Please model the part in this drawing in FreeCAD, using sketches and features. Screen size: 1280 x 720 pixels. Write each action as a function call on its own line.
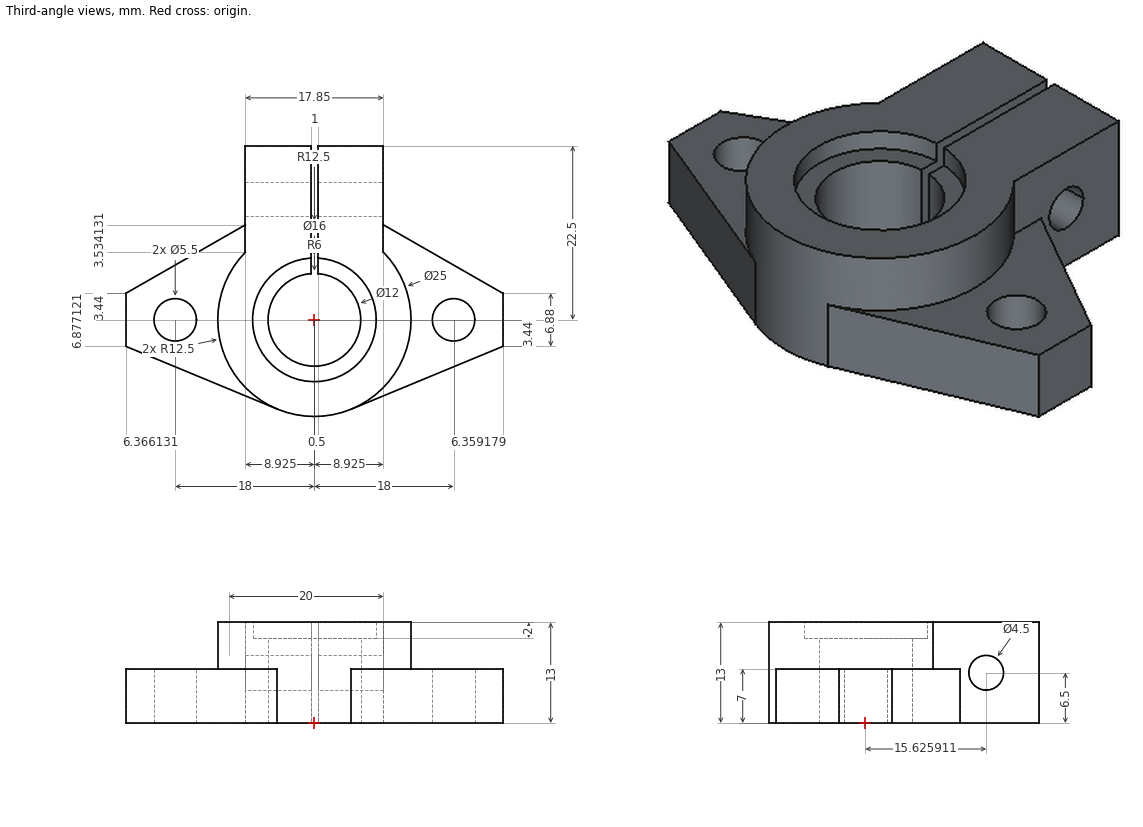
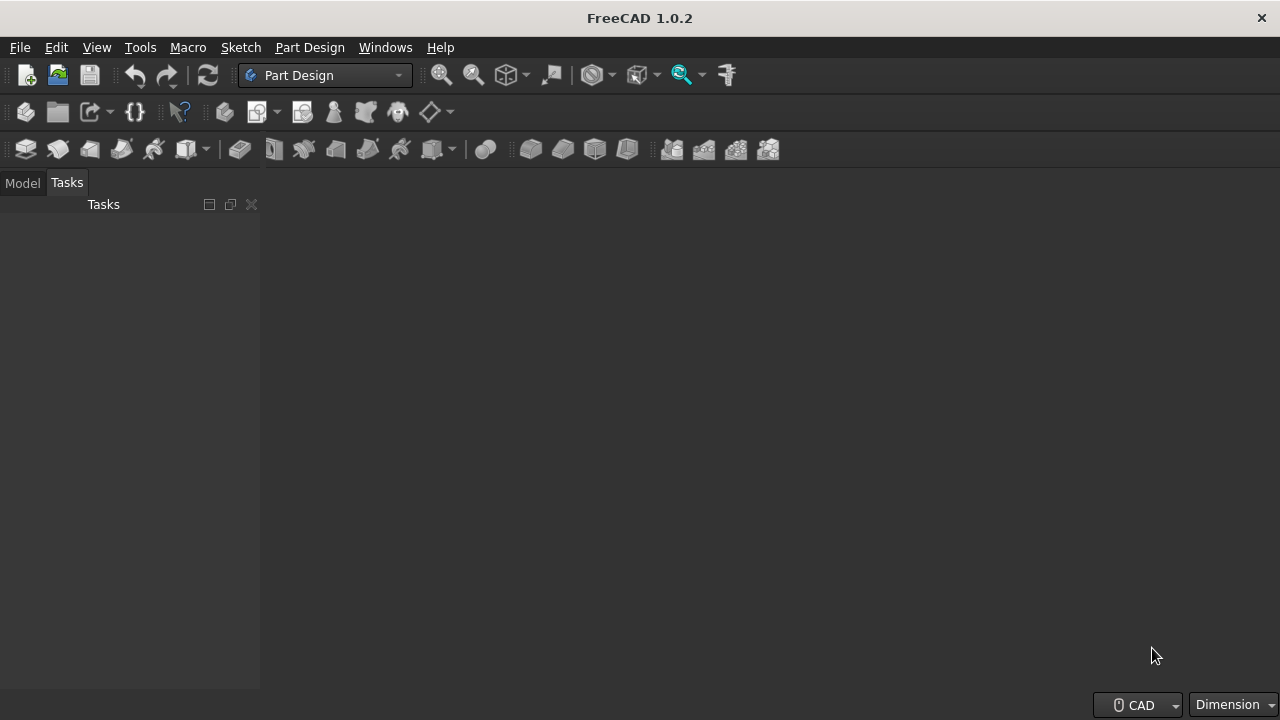
click(26, 76)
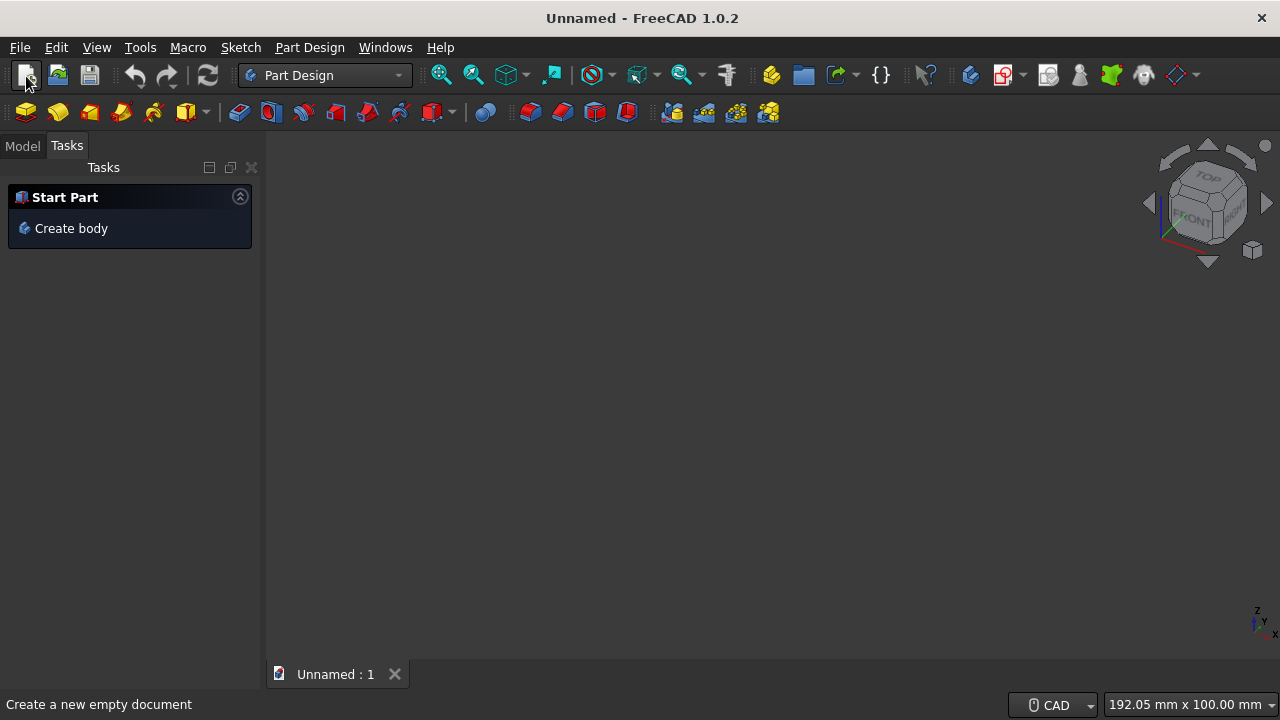
click(1004, 76)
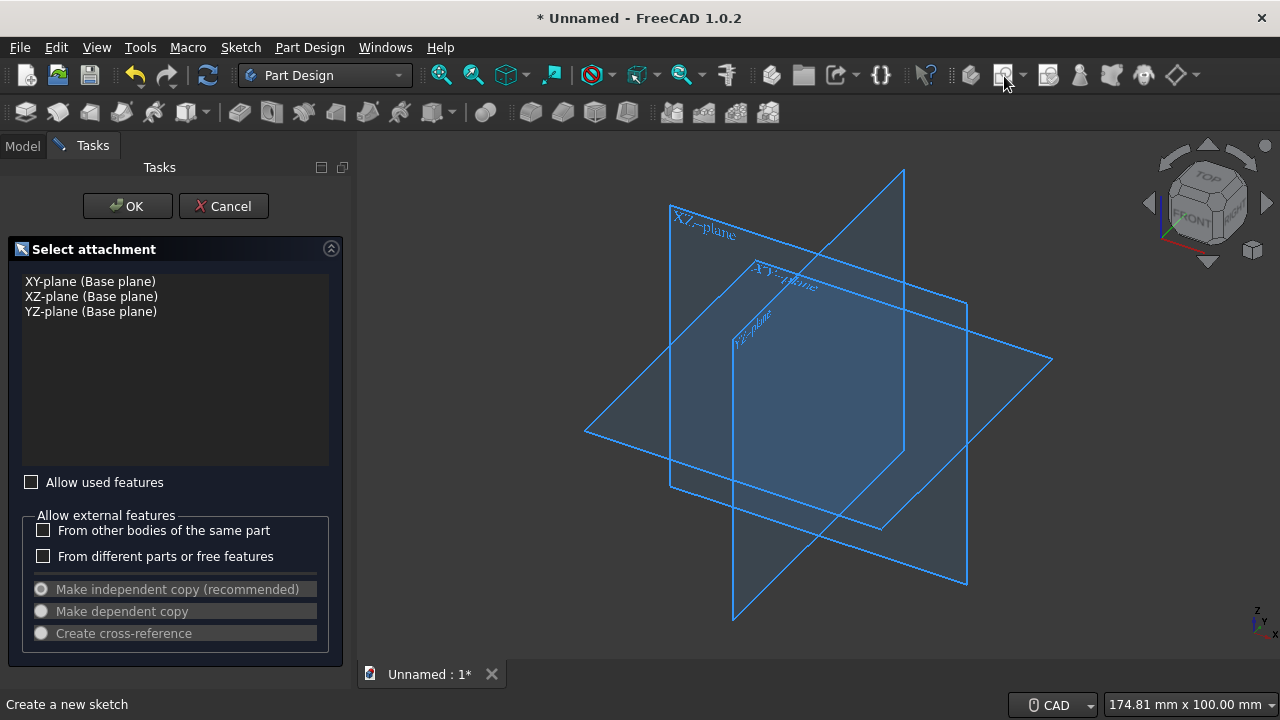
click(82, 282)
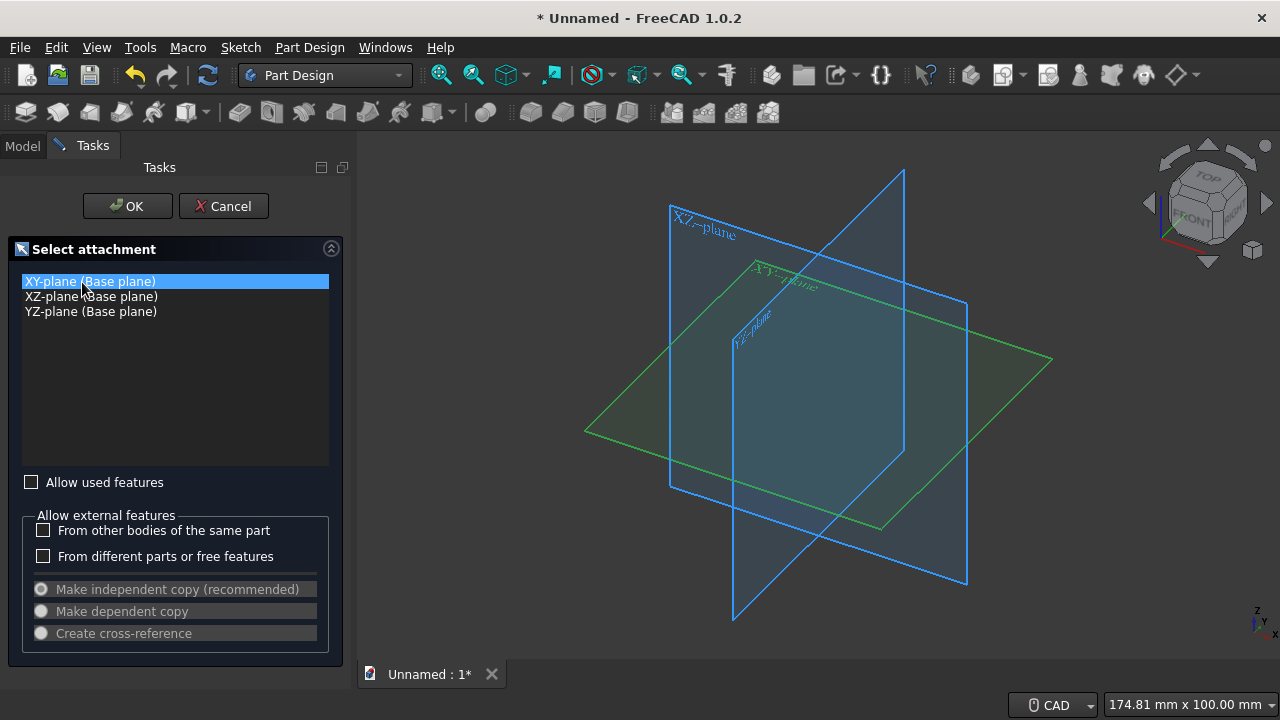
click(128, 206)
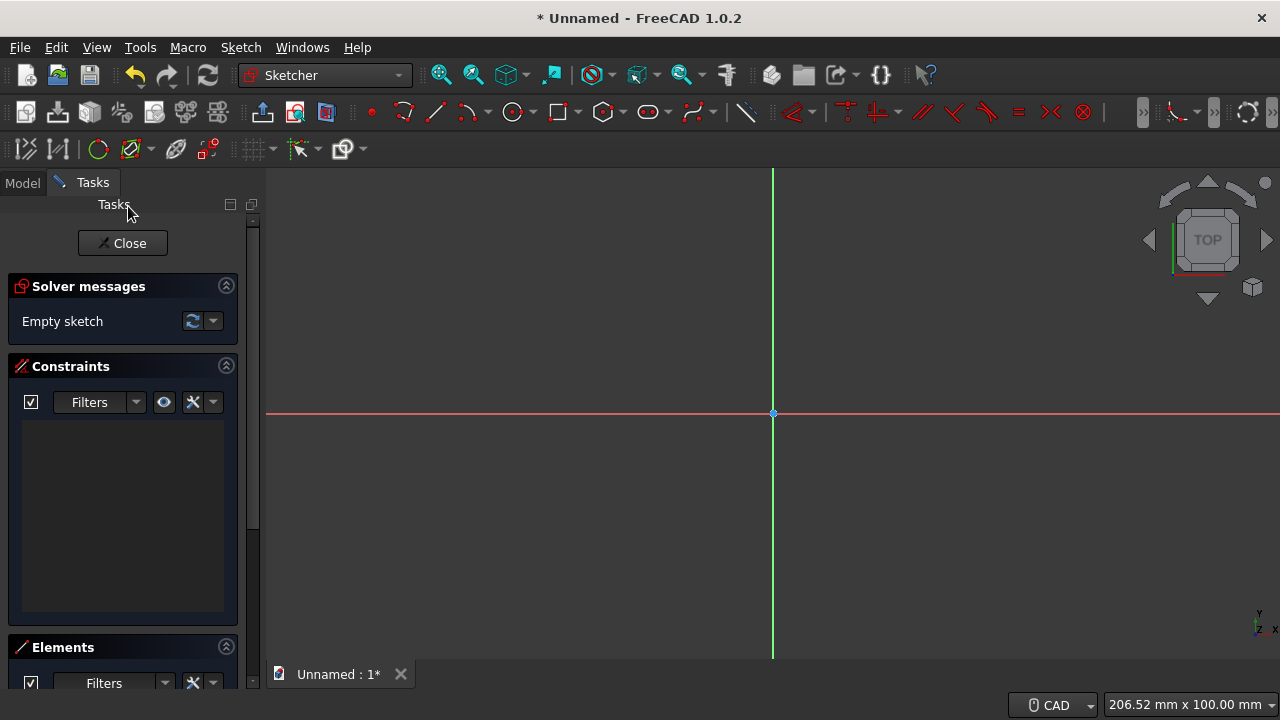
scroll(813, 414, up, 5)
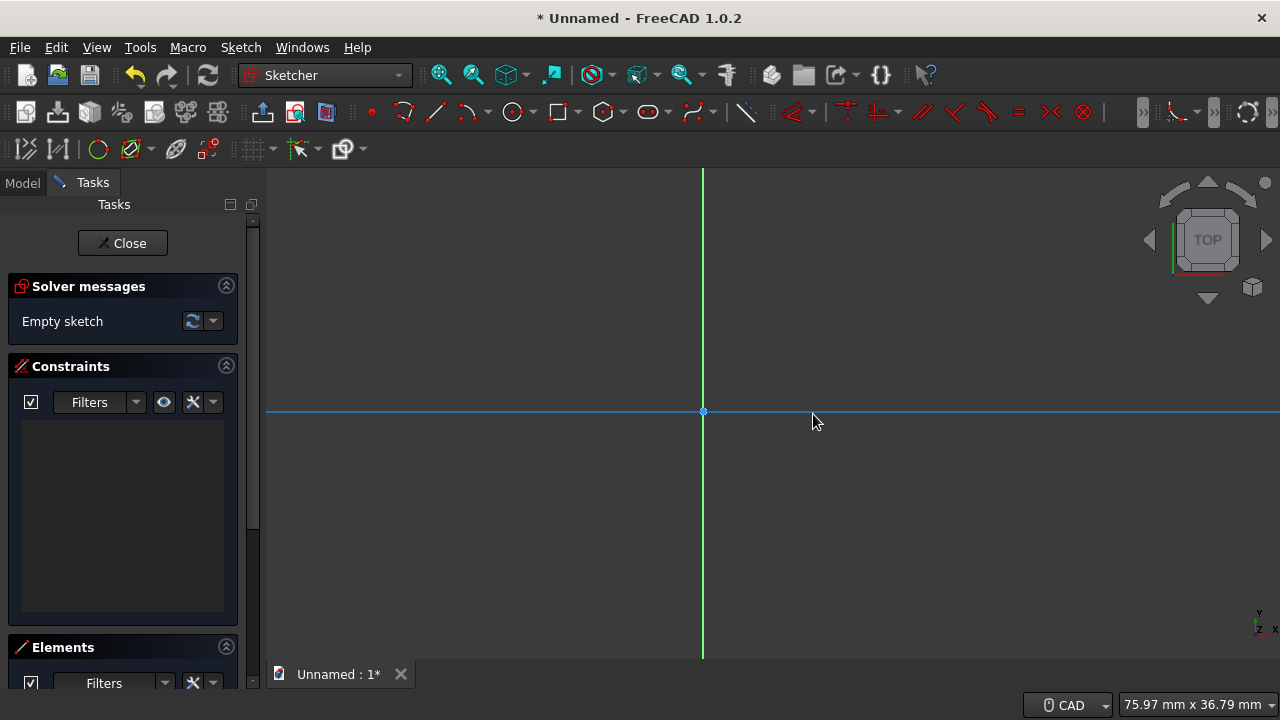
click(514, 112)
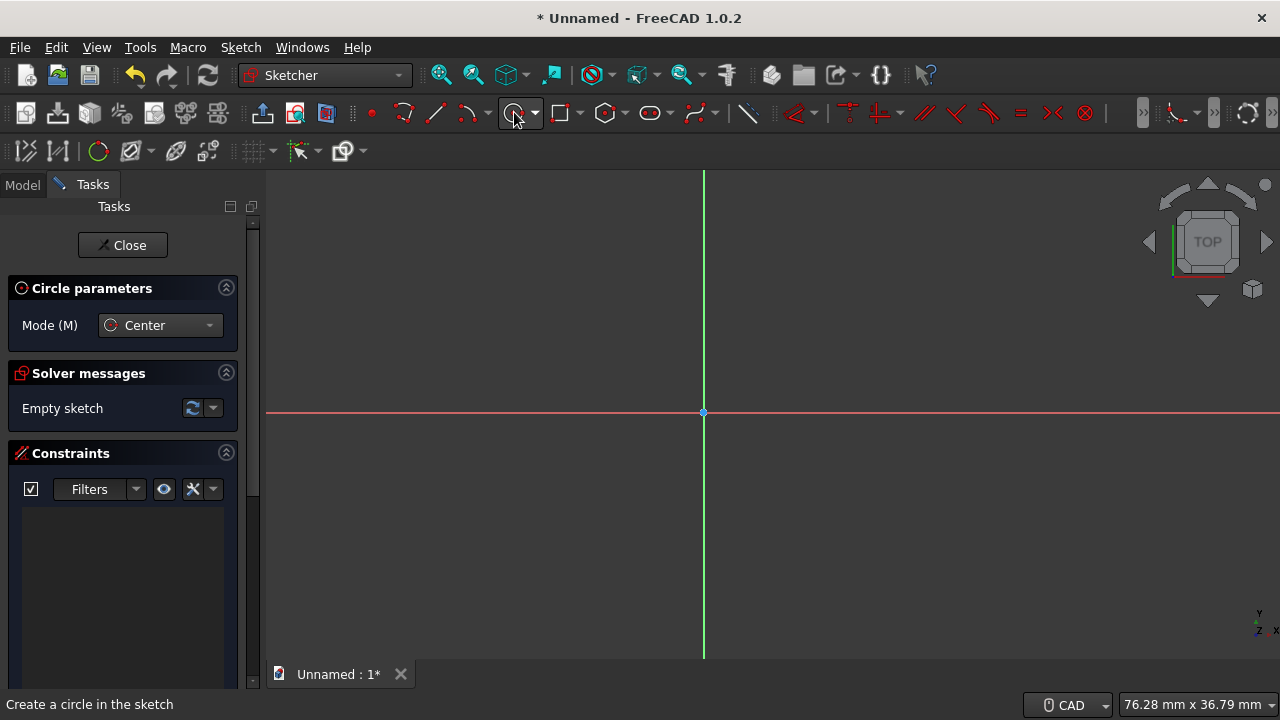
click(704, 413)
click(821, 295)
key(Escape)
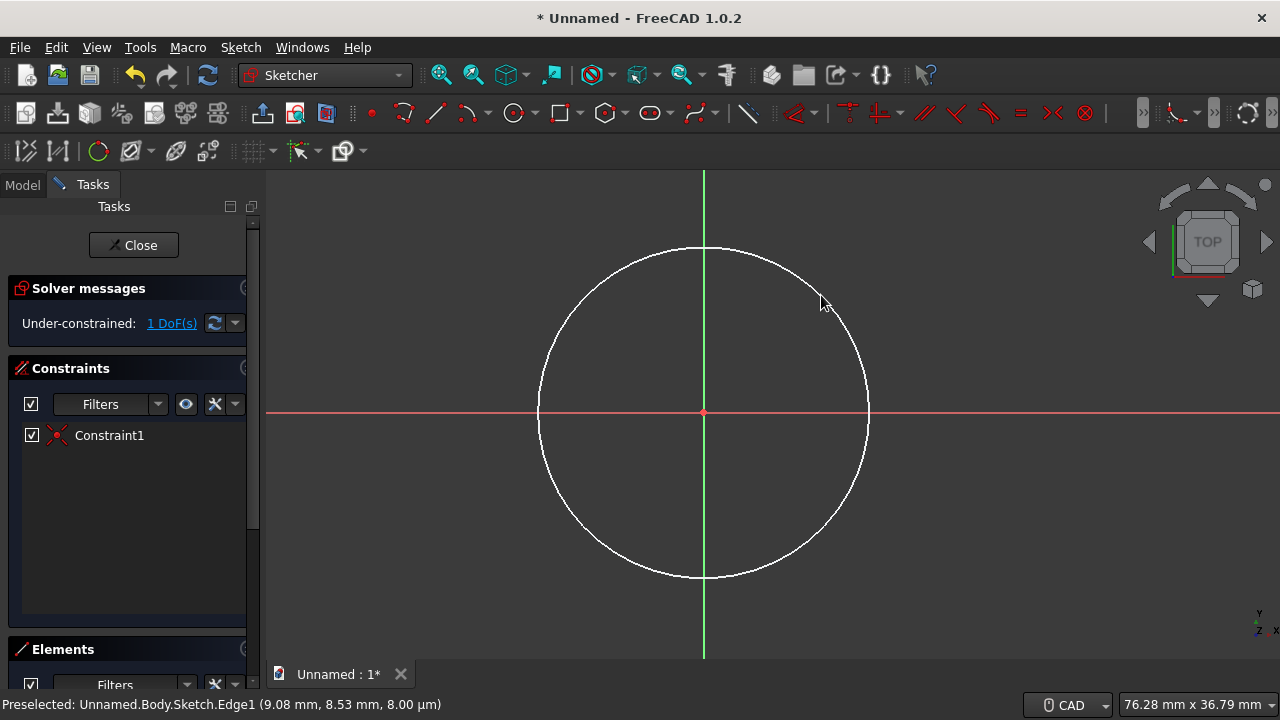
click(820, 295)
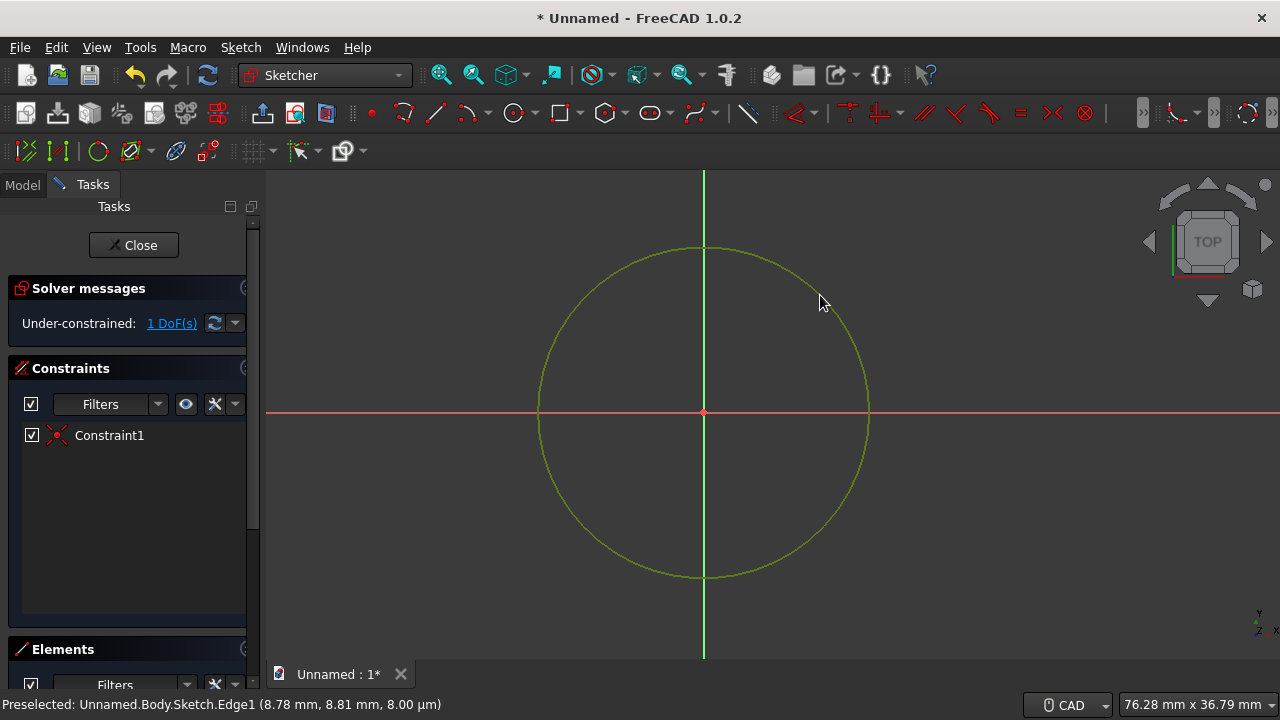
click(816, 114)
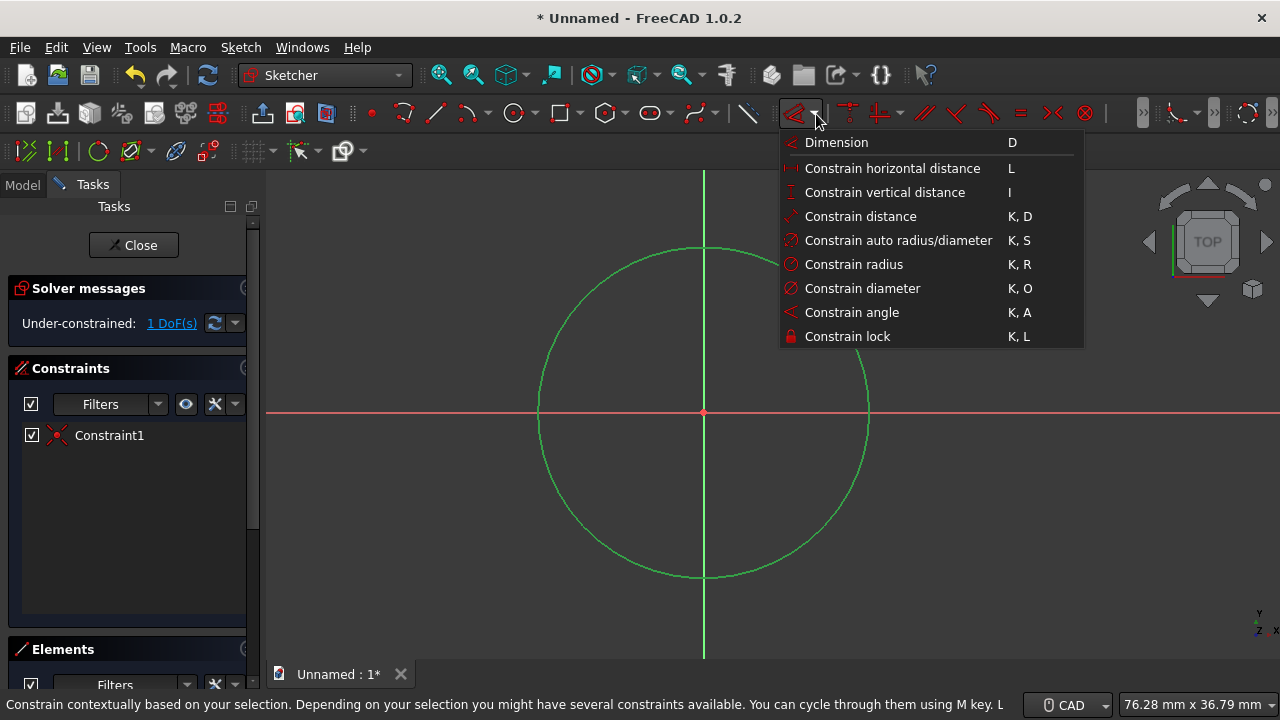
click(932, 288)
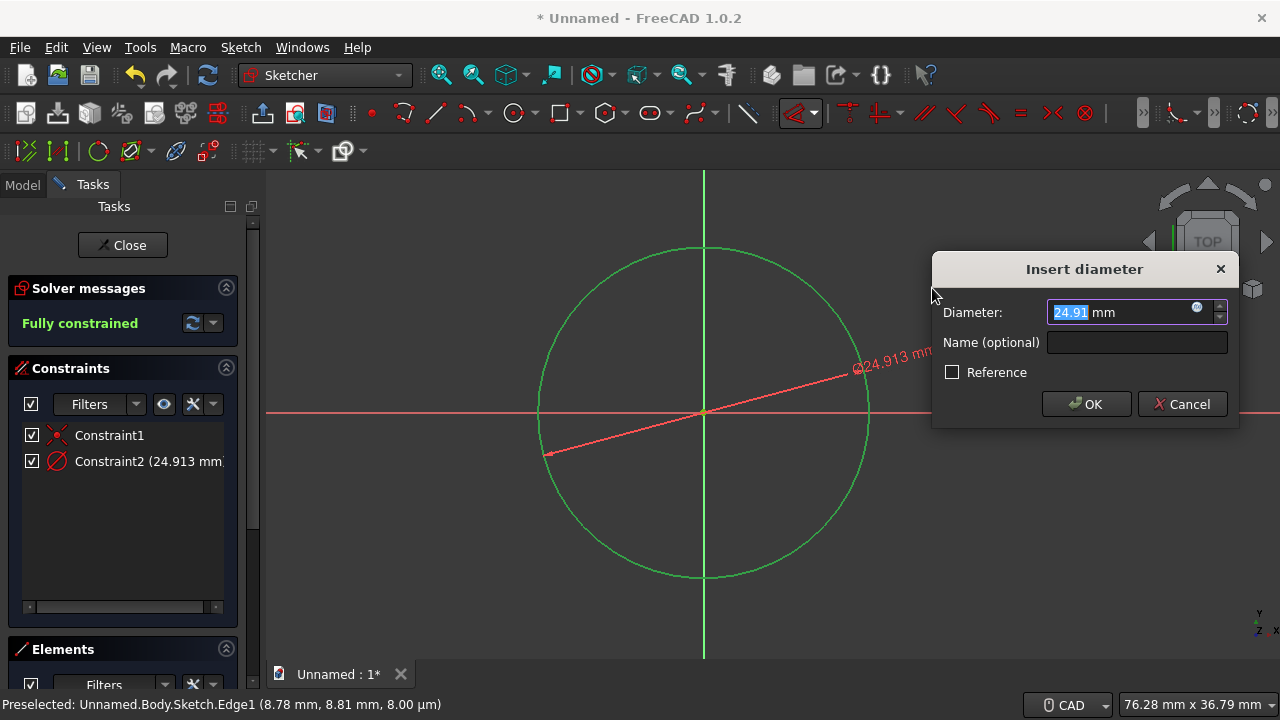
text(25)
key(Return)